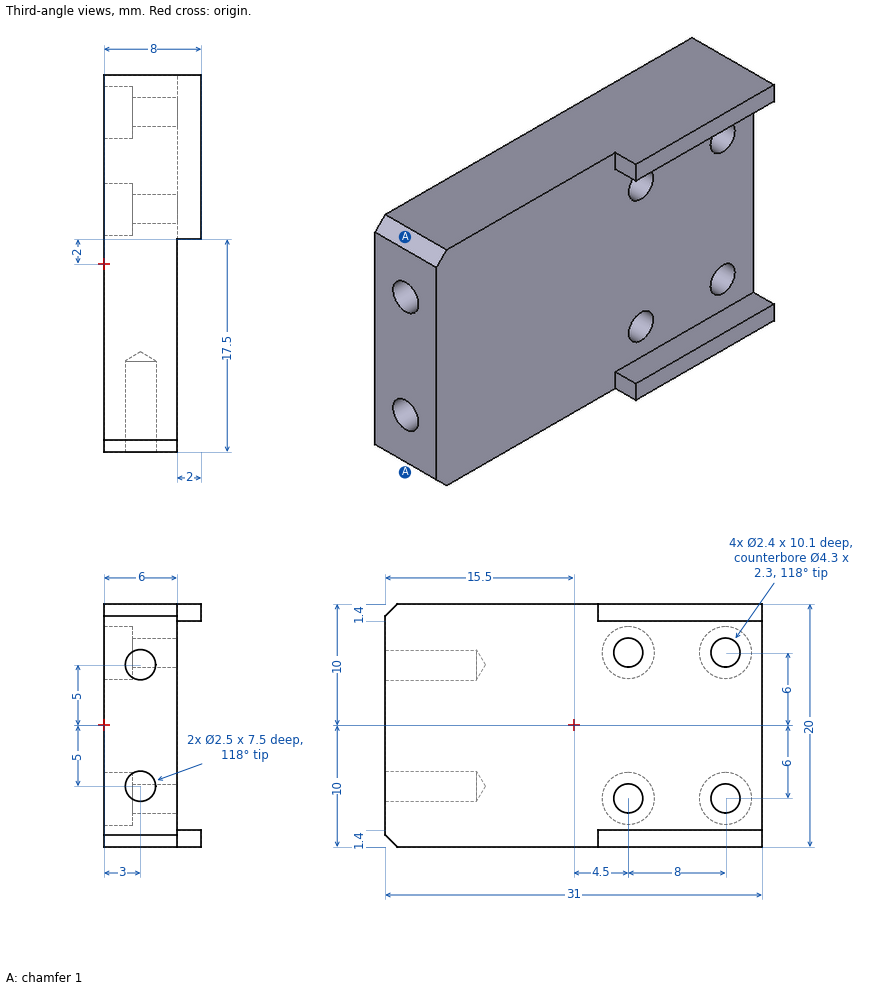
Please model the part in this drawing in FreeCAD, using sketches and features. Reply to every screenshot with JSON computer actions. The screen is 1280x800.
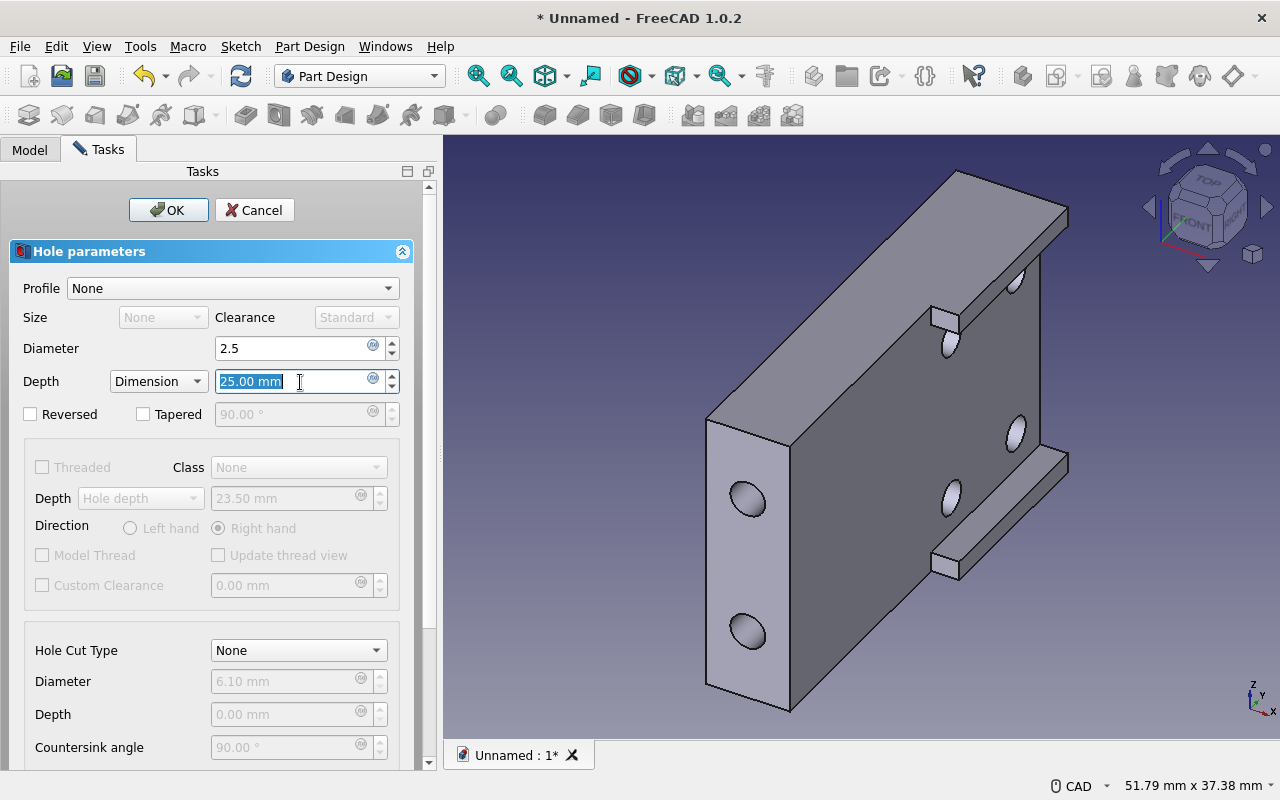
{"action": "type", "text": "7.5"}
{"action": "key", "text": "Tab"}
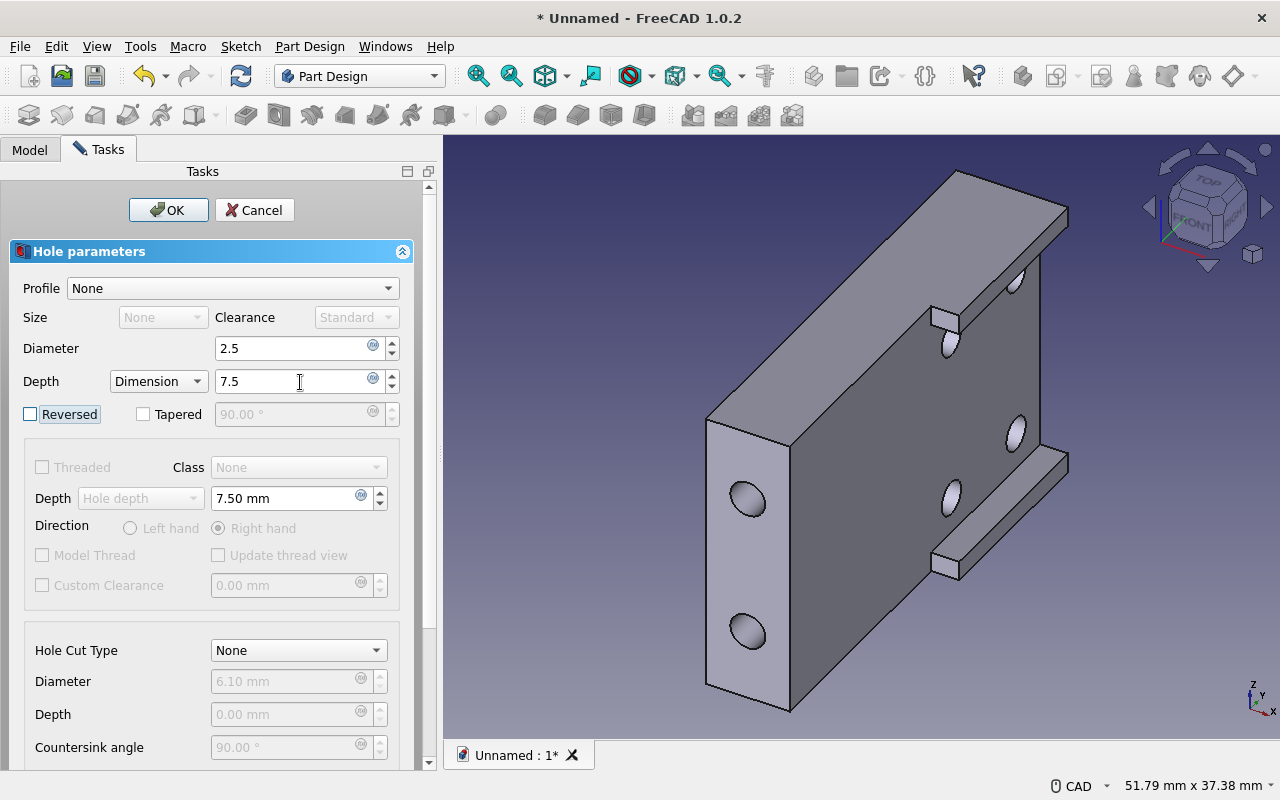
{"action": "left_click", "coordinate": [169, 210]}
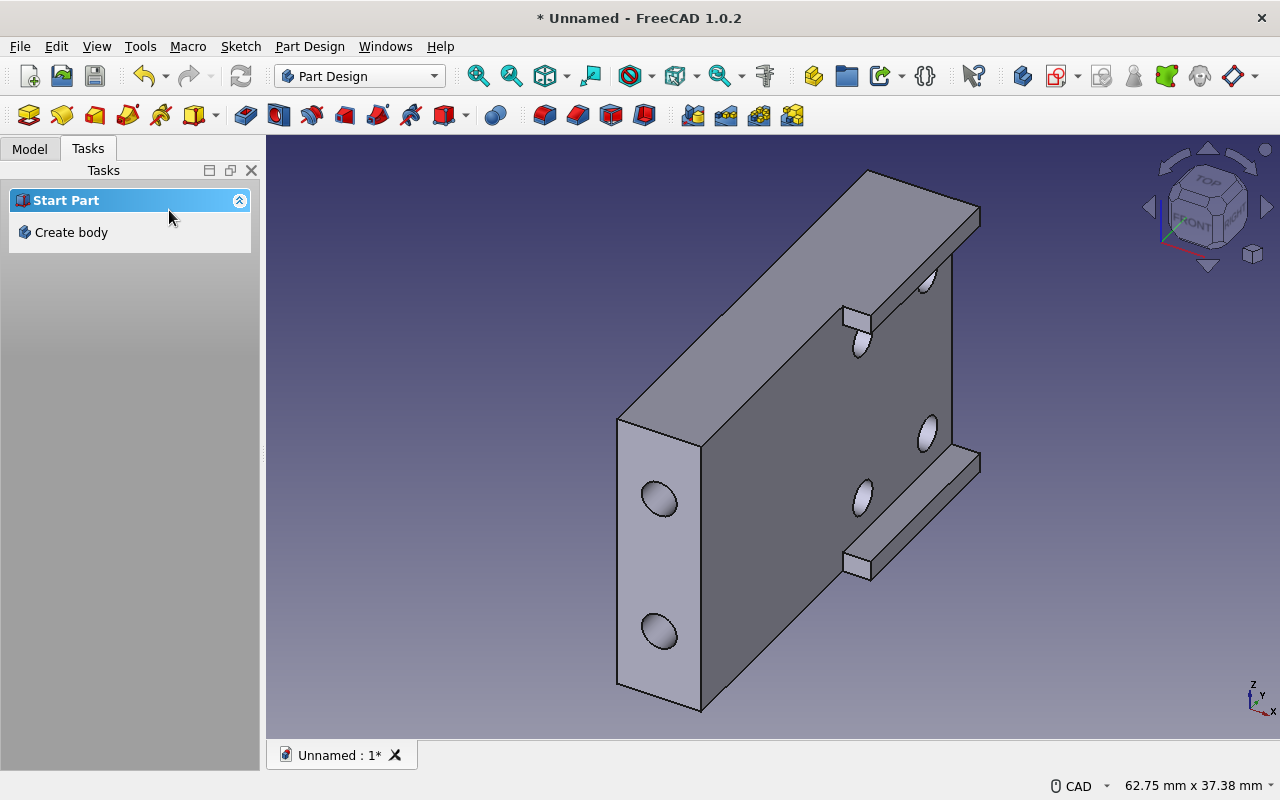
{"action": "left_click", "coordinate": [659, 432]}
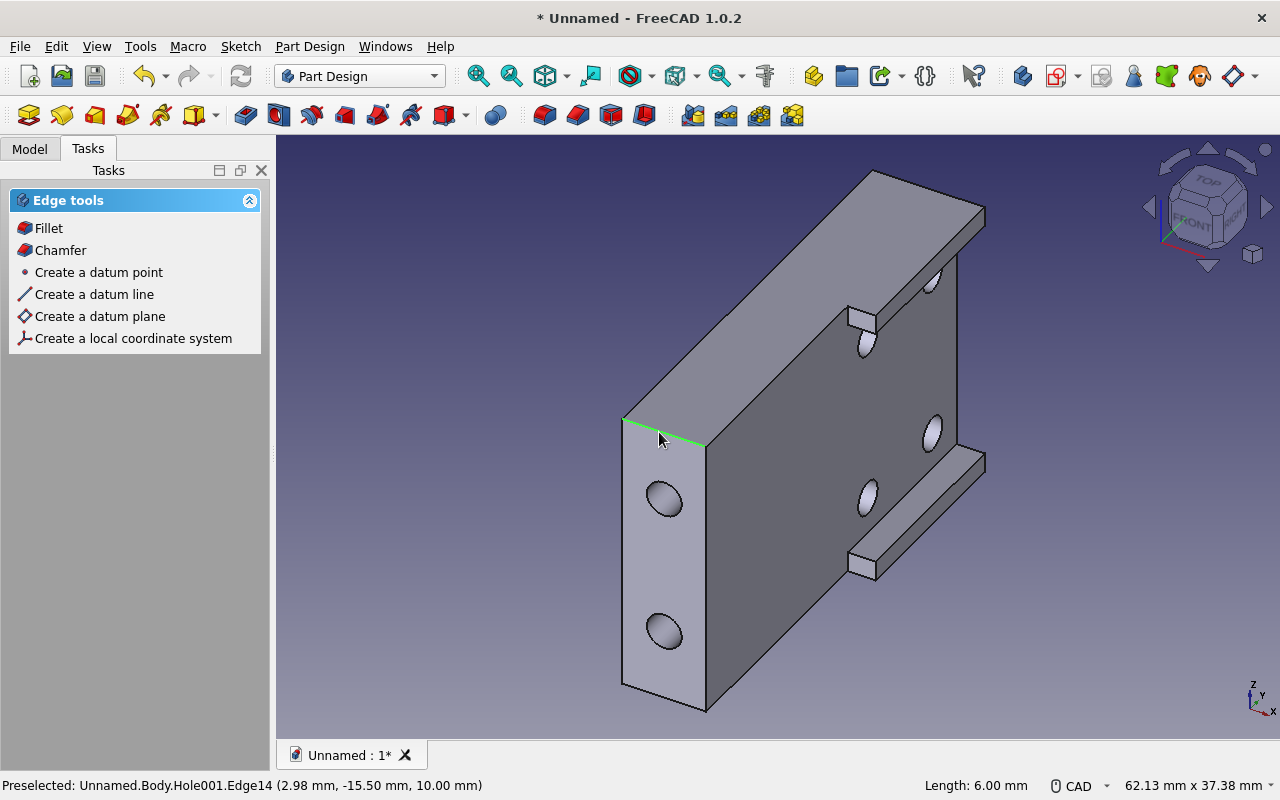
{"action": "key", "text": "0"}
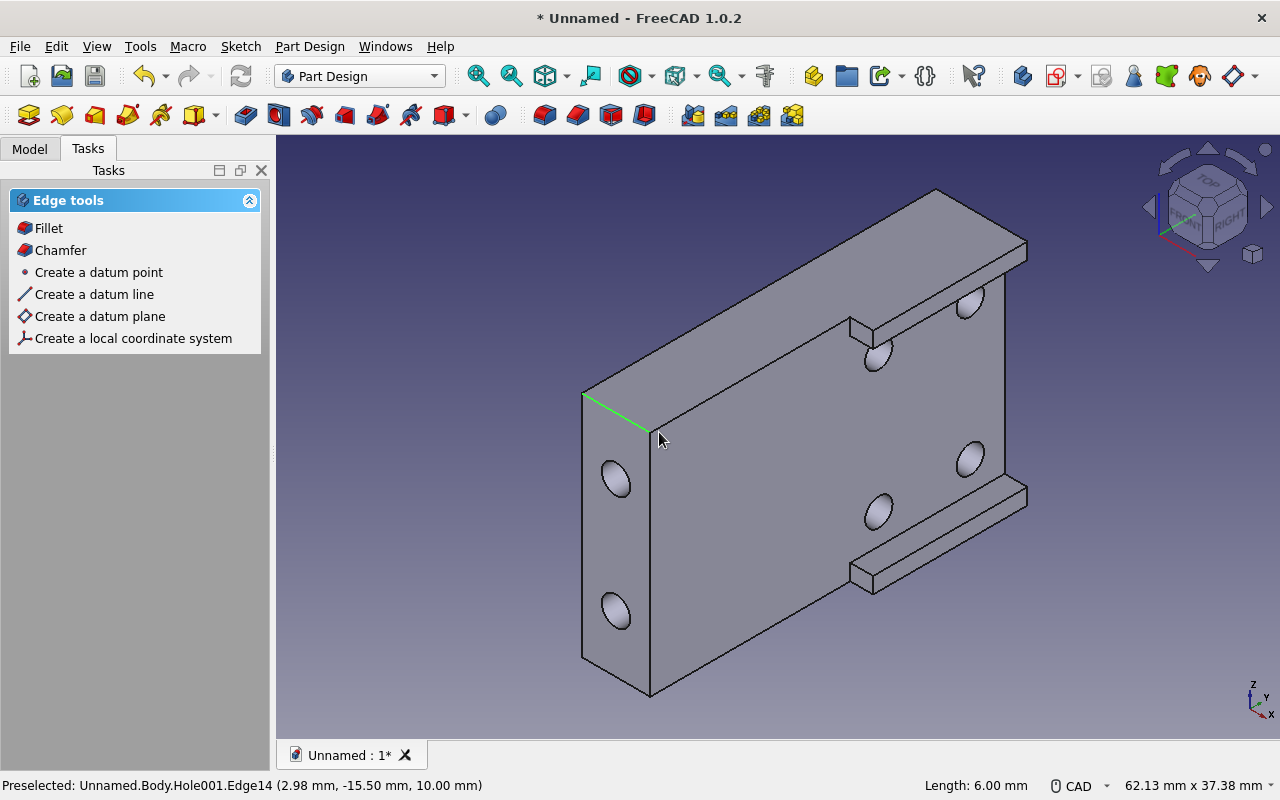
{"action": "key", "text": "2"}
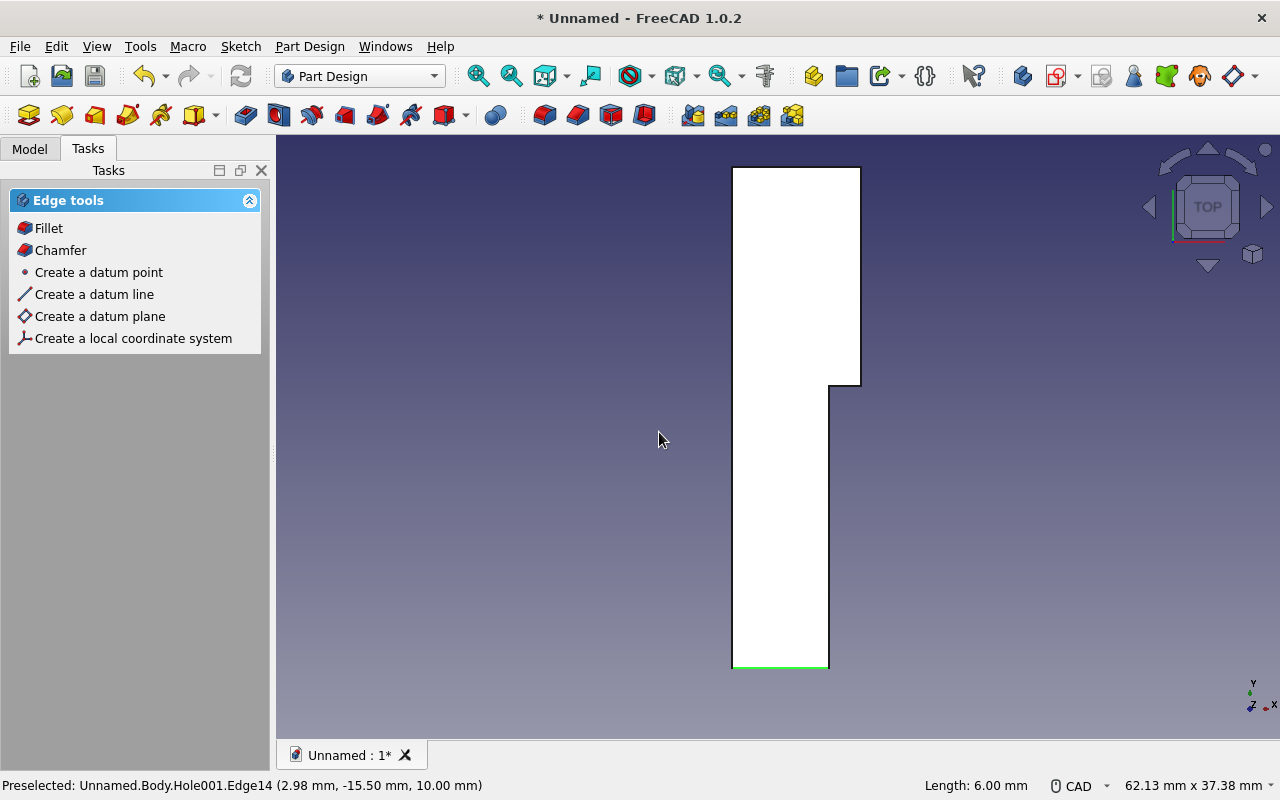
{"action": "key", "text": "1"}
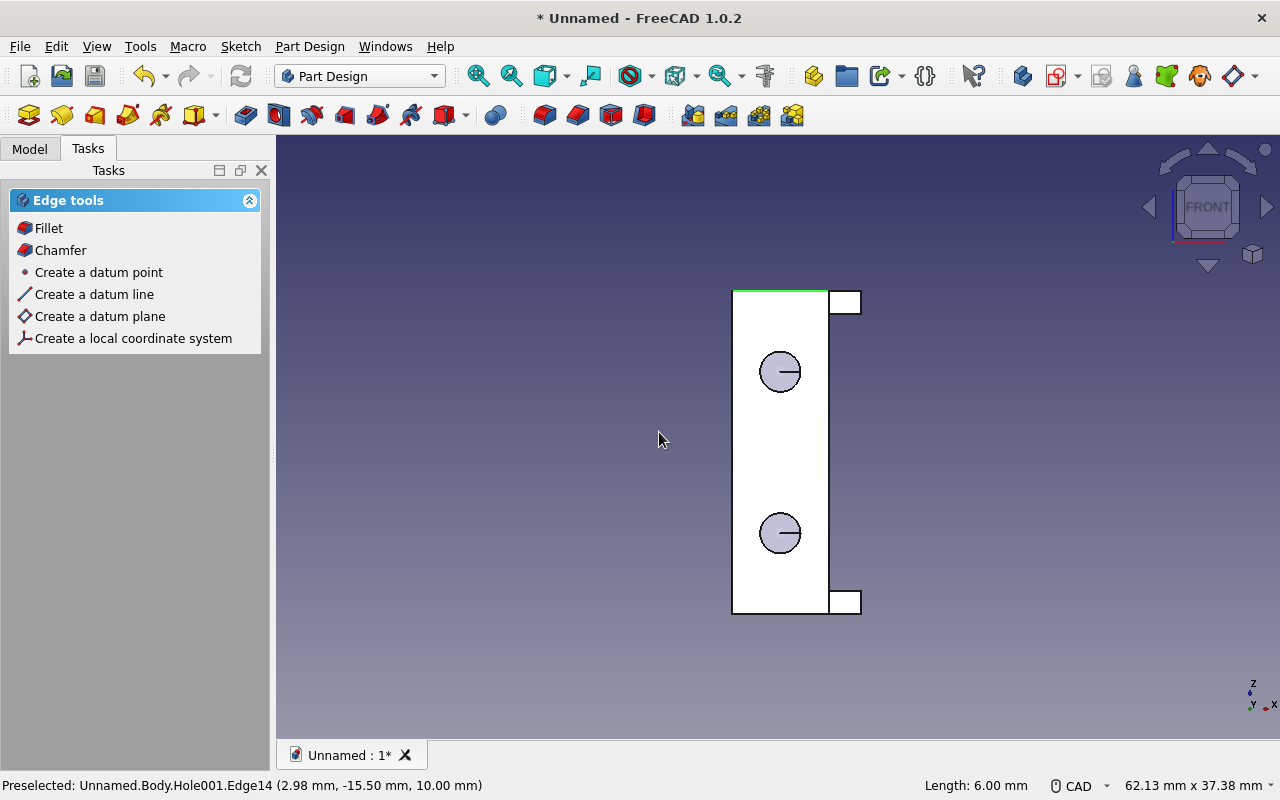
{"action": "left_click", "coordinate": [780, 613], "text": "ctrl"}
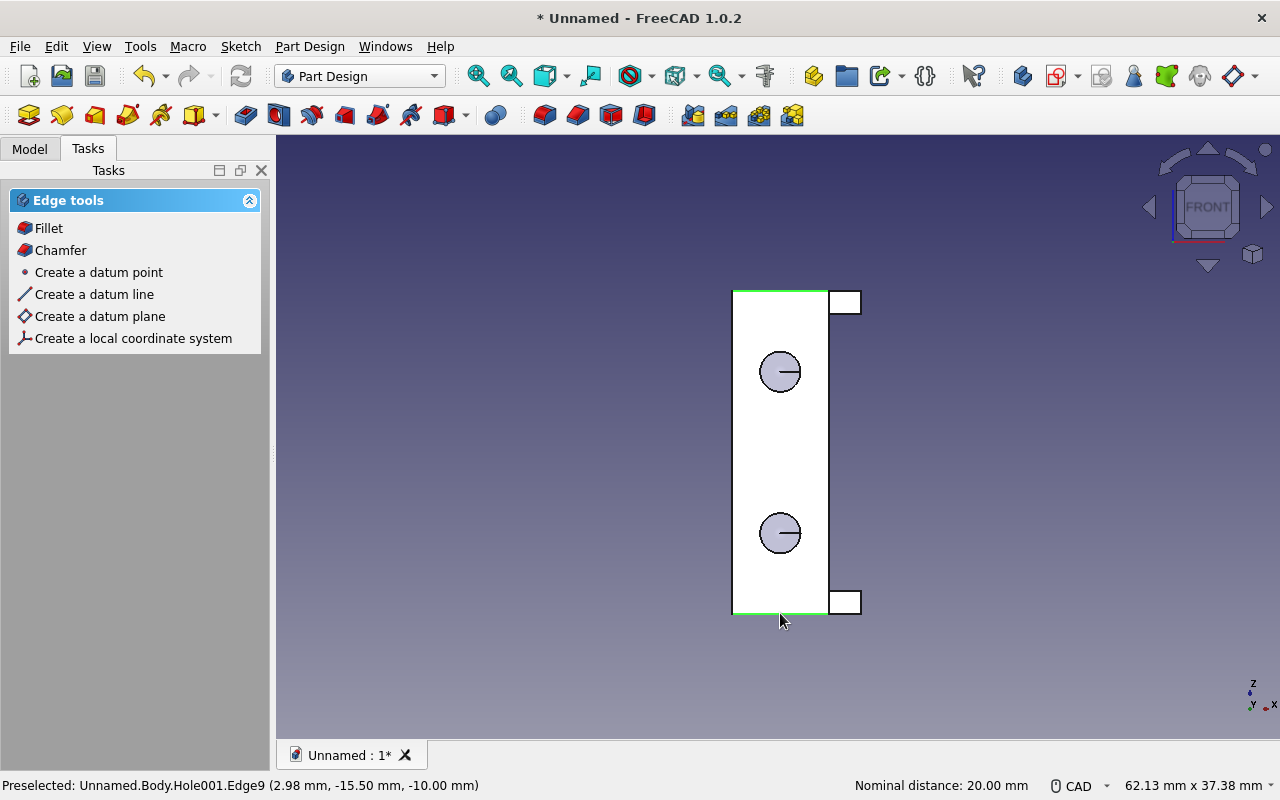
{"action": "left_click", "coordinate": [578, 116]}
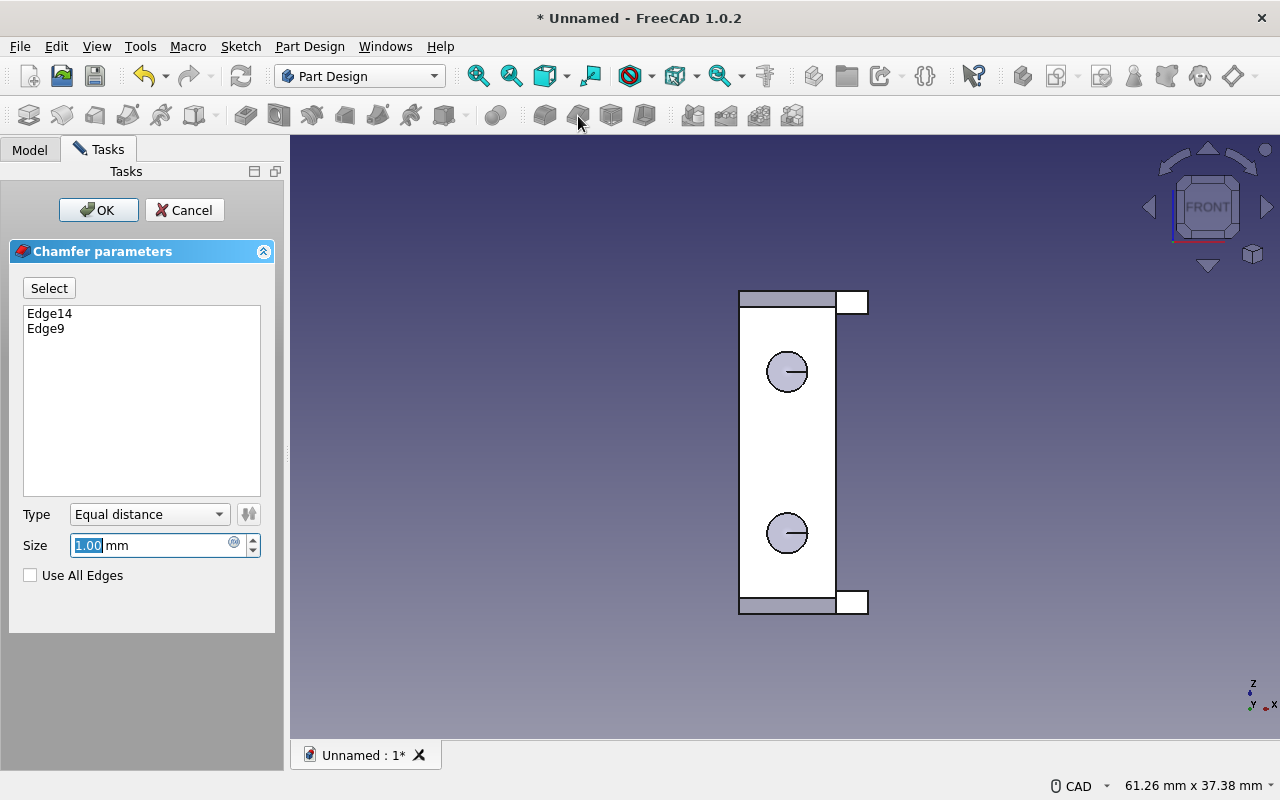
{"action": "type", "text": "1"}
{"action": "key", "text": "Tab"}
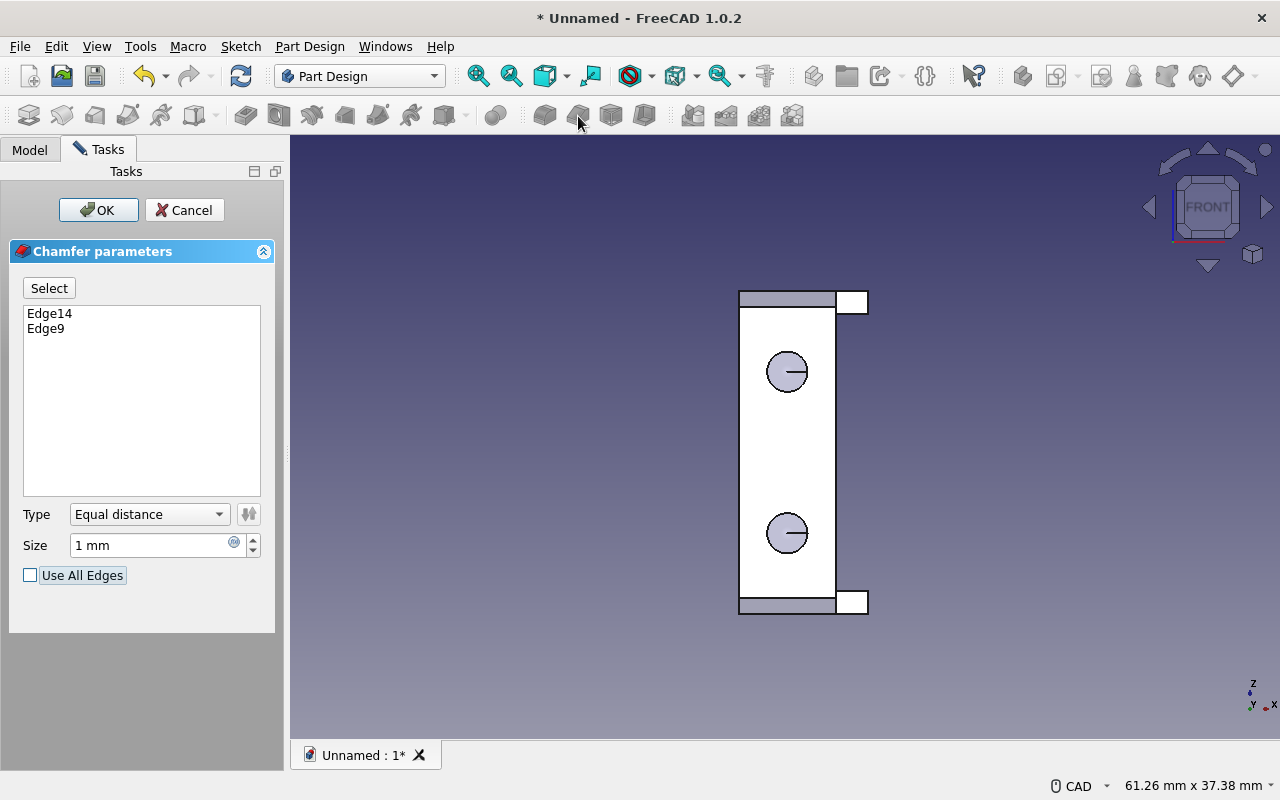
{"action": "left_click", "coordinate": [99, 210]}